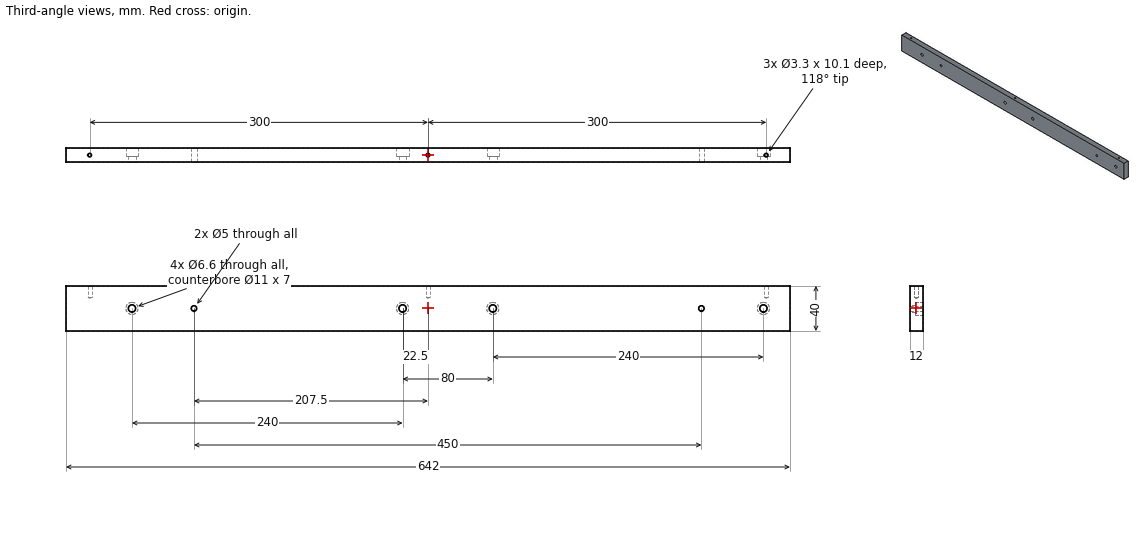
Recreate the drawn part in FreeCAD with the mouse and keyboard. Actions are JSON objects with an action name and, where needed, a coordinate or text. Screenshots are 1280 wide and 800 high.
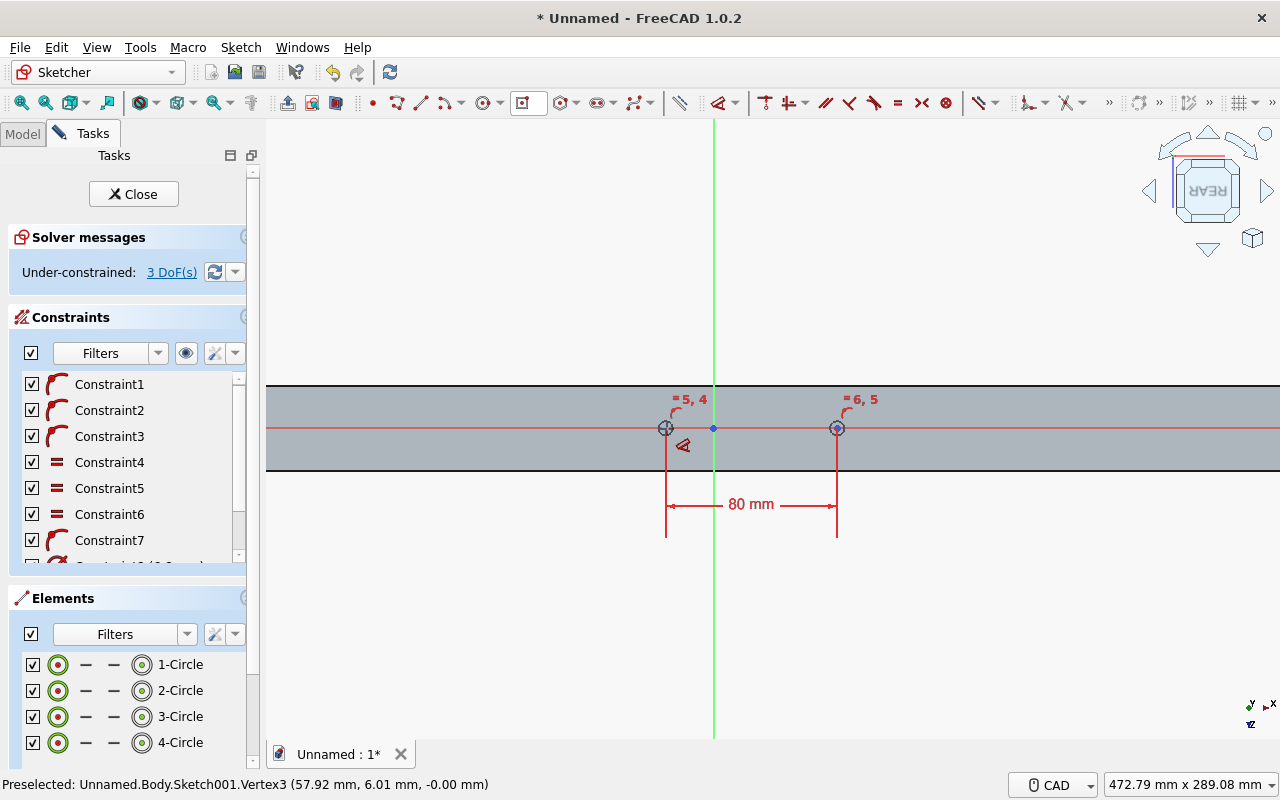
{"action": "left_click", "coordinate": [666, 428]}
{"action": "left_click", "coordinate": [690, 462]}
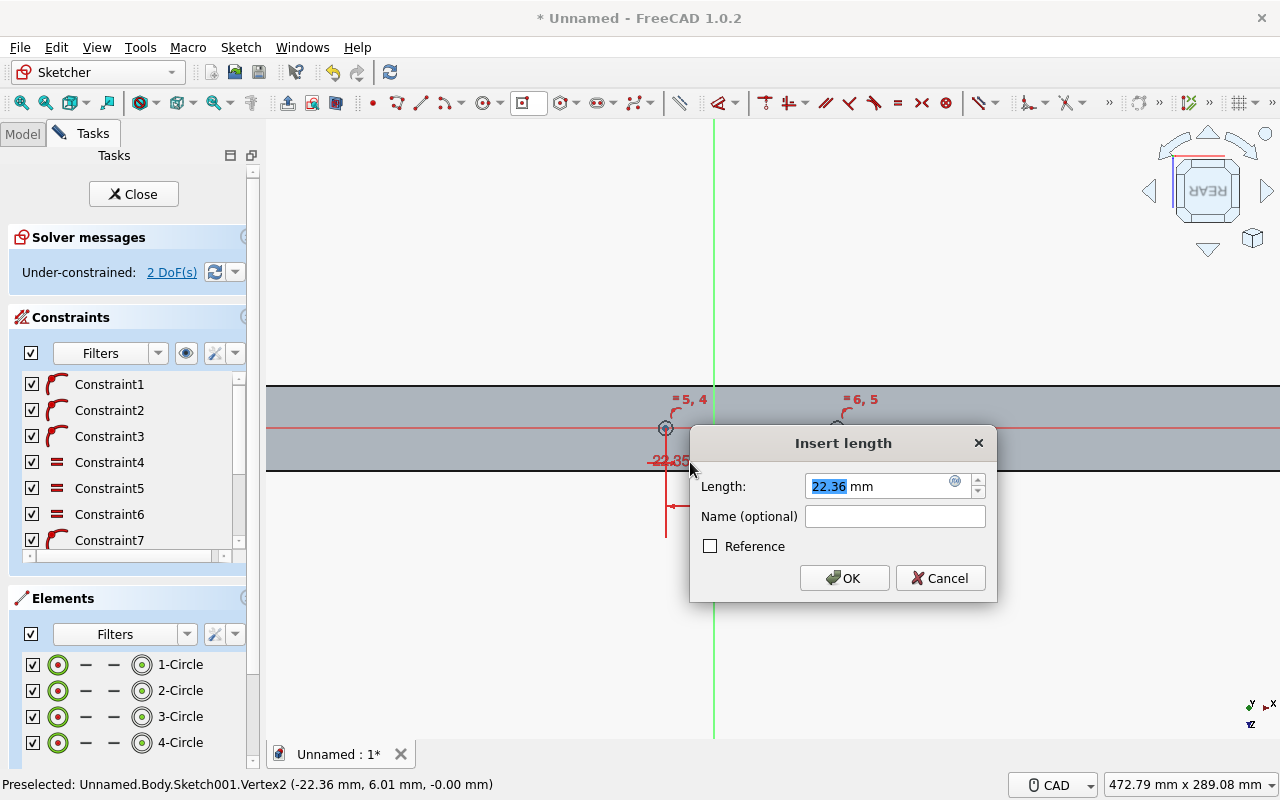
{"action": "type", "text": "22.5"}
{"action": "key", "text": "Return"}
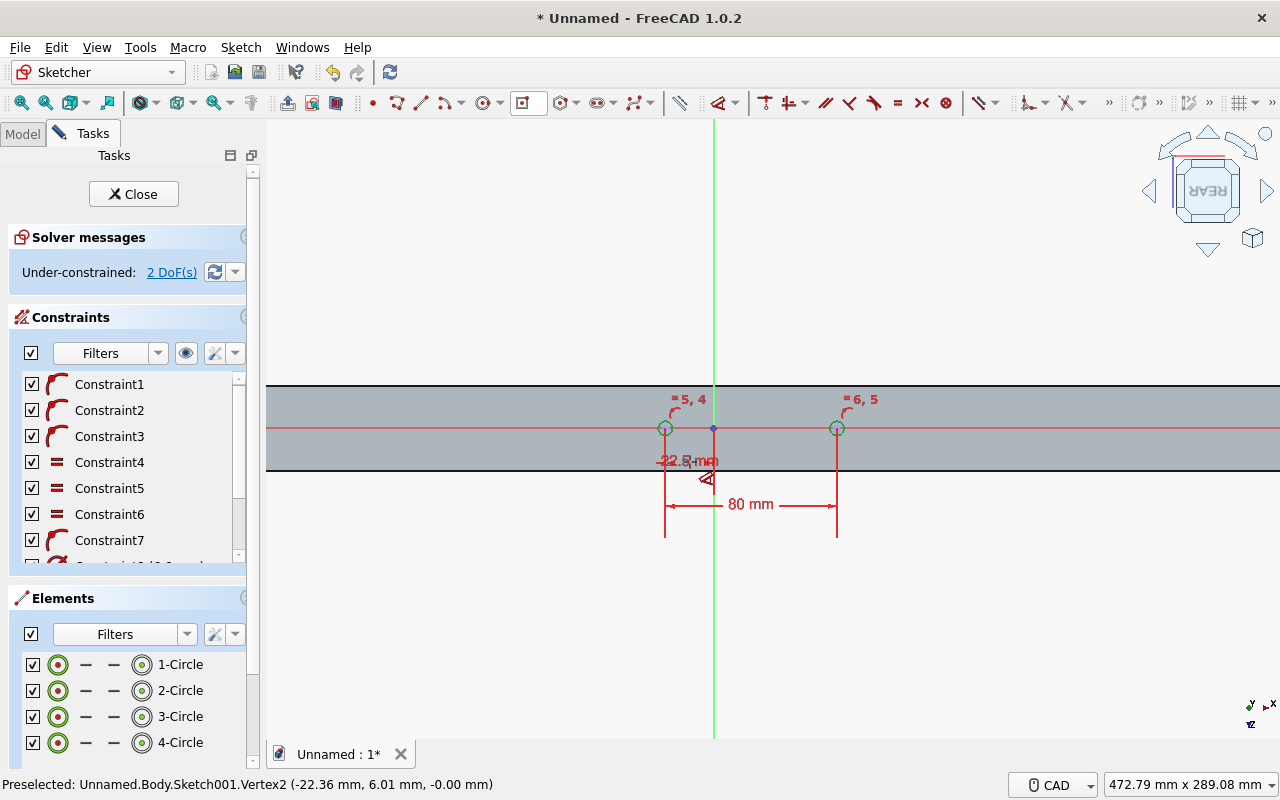
{"action": "scroll", "coordinate": [666, 429], "scroll_direction": "down", "scroll_amount": 4}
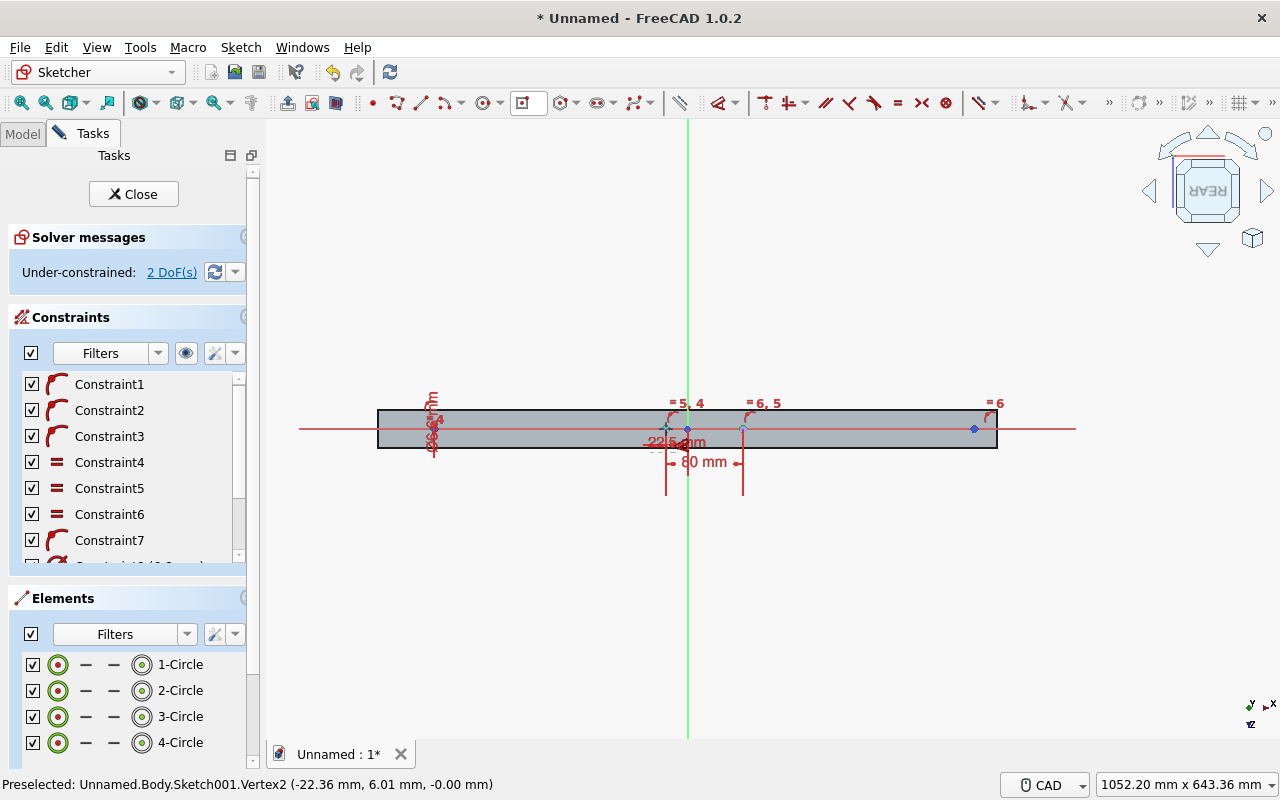
{"action": "left_click", "coordinate": [434, 429]}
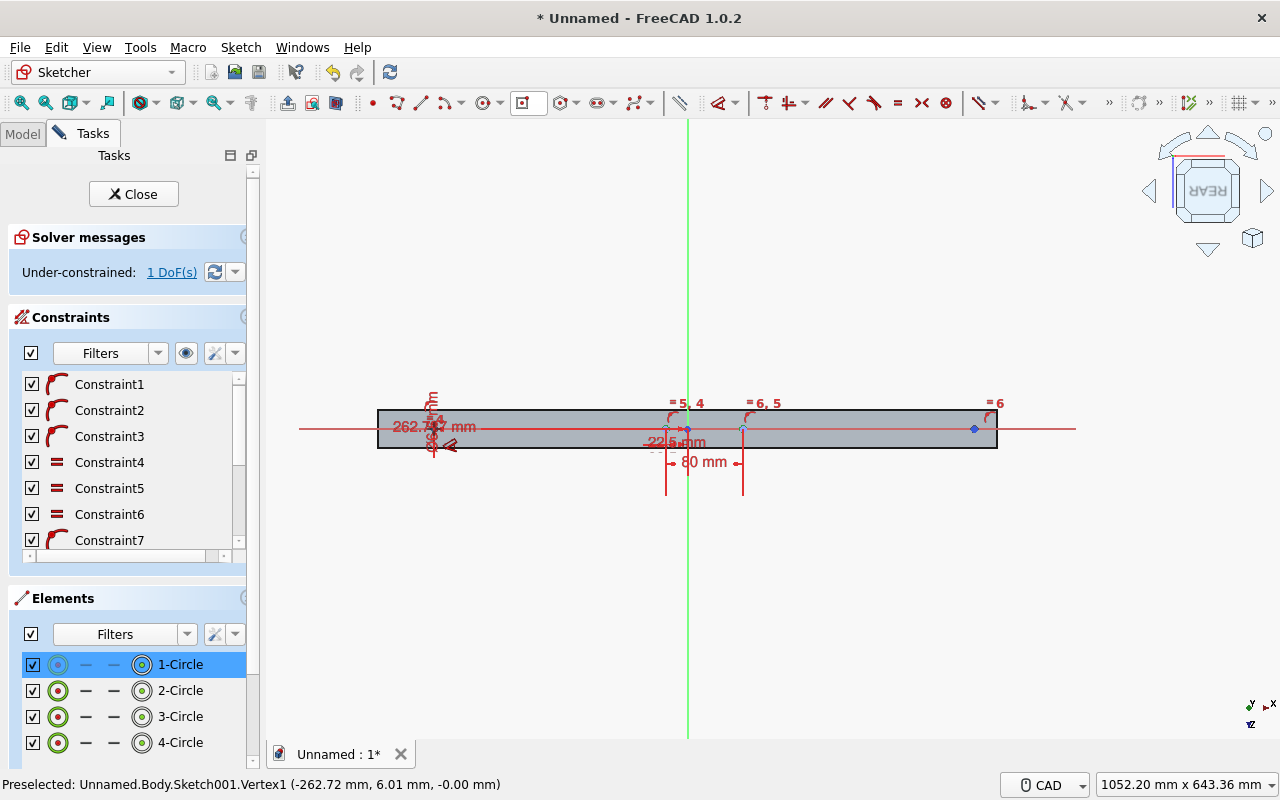
{"action": "left_click", "coordinate": [666, 429]}
{"action": "left_click", "coordinate": [550, 463]}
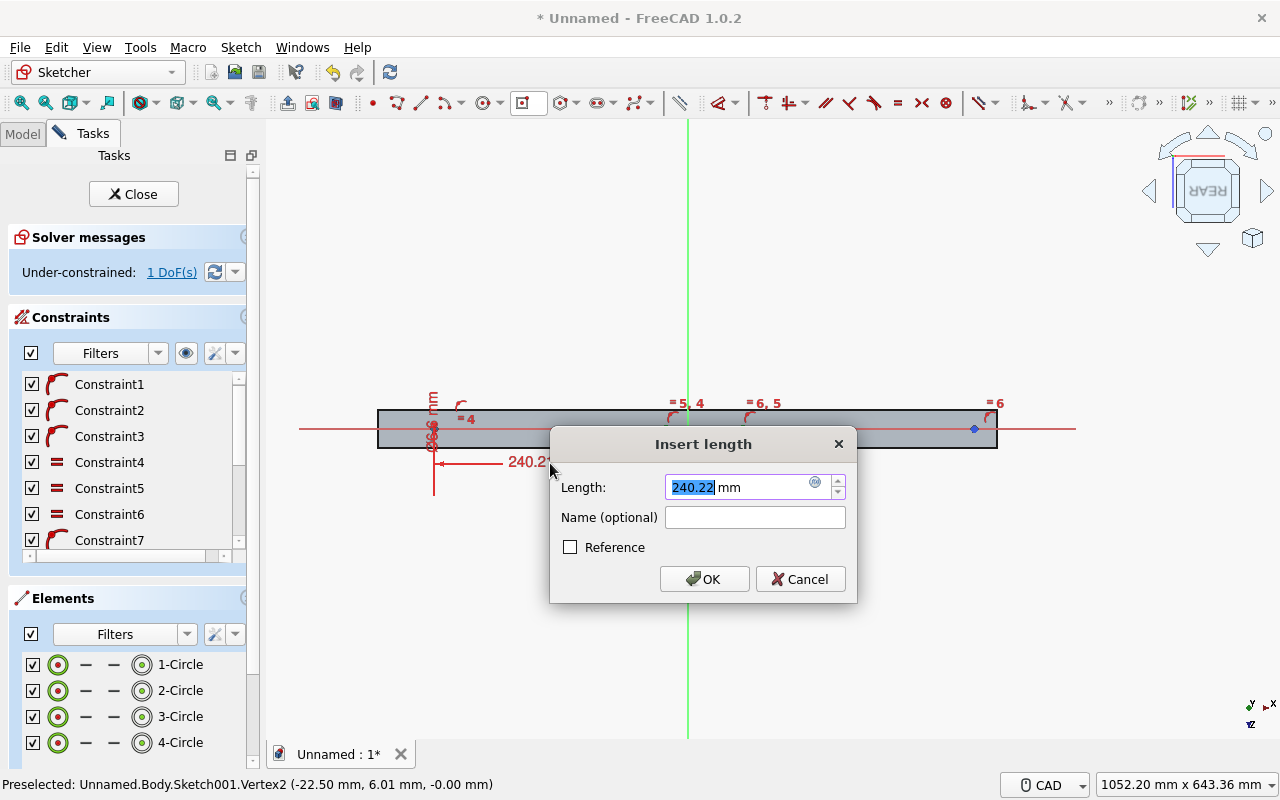
{"action": "type", "text": "240"}
{"action": "key", "text": "Return"}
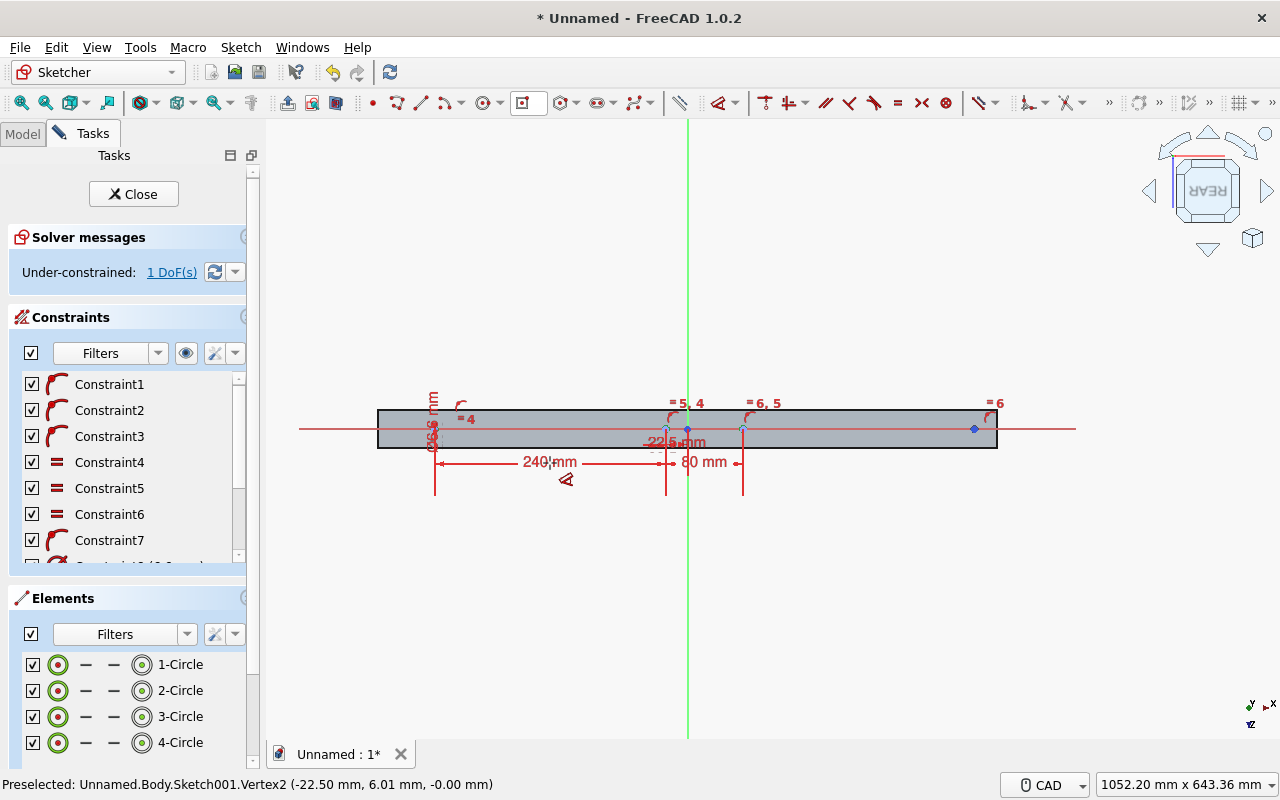
{"action": "left_click", "coordinate": [743, 429]}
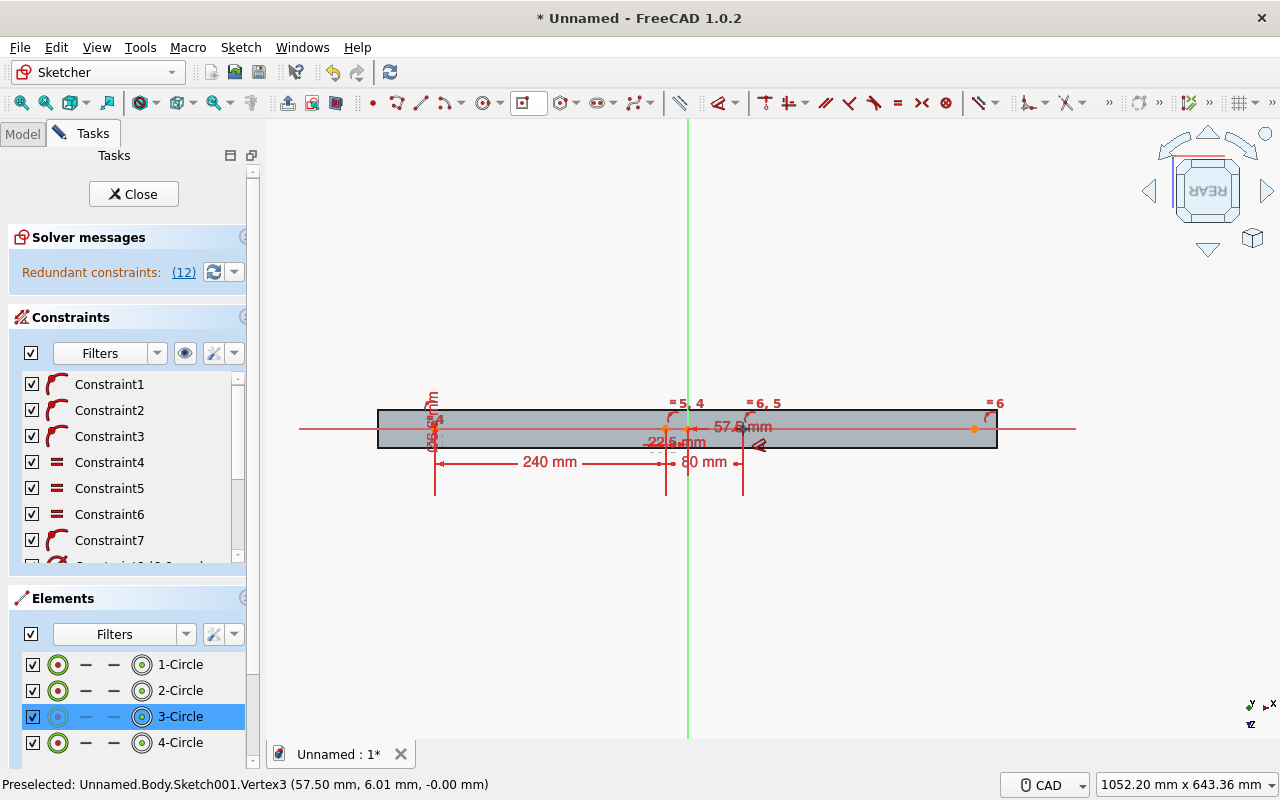
{"action": "left_click", "coordinate": [974, 429]}
{"action": "left_click", "coordinate": [859, 463]}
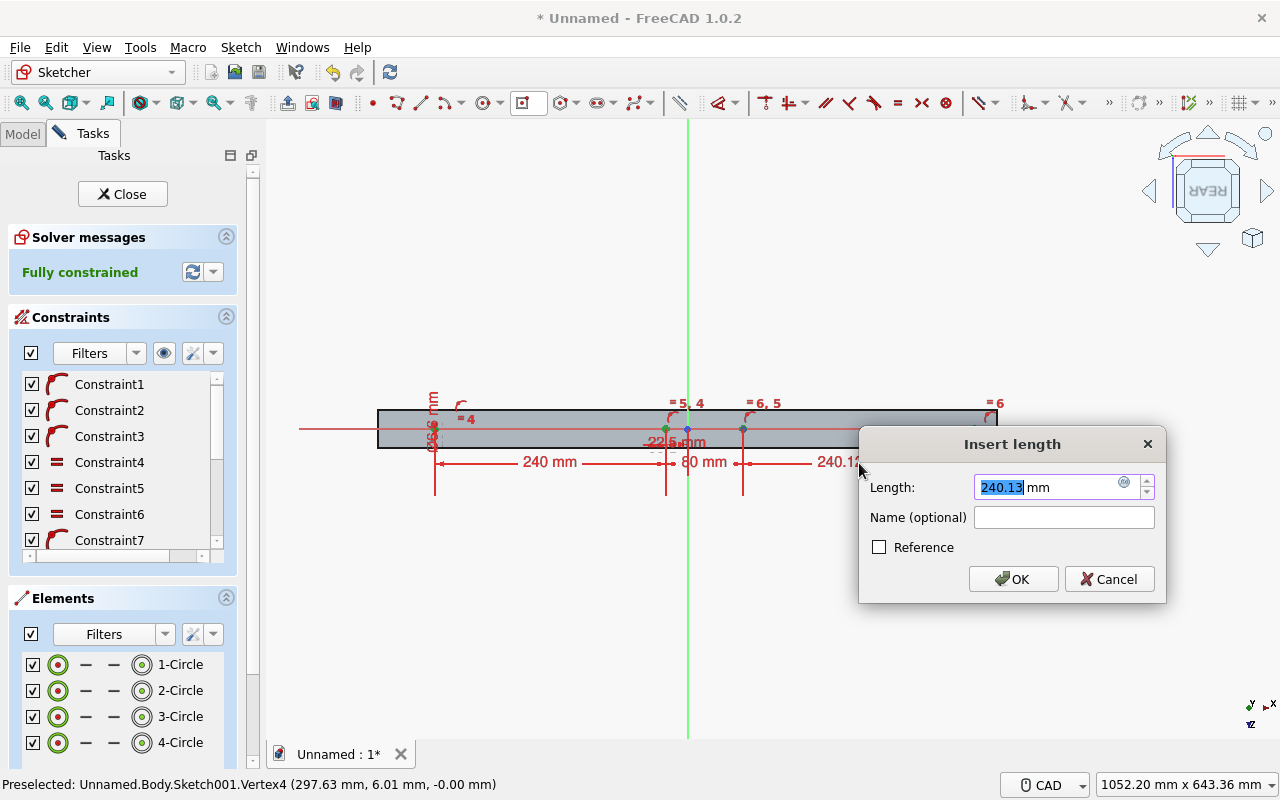
{"action": "type", "text": "240"}
{"action": "key", "text": "Return"}
{"action": "key", "text": "Escape"}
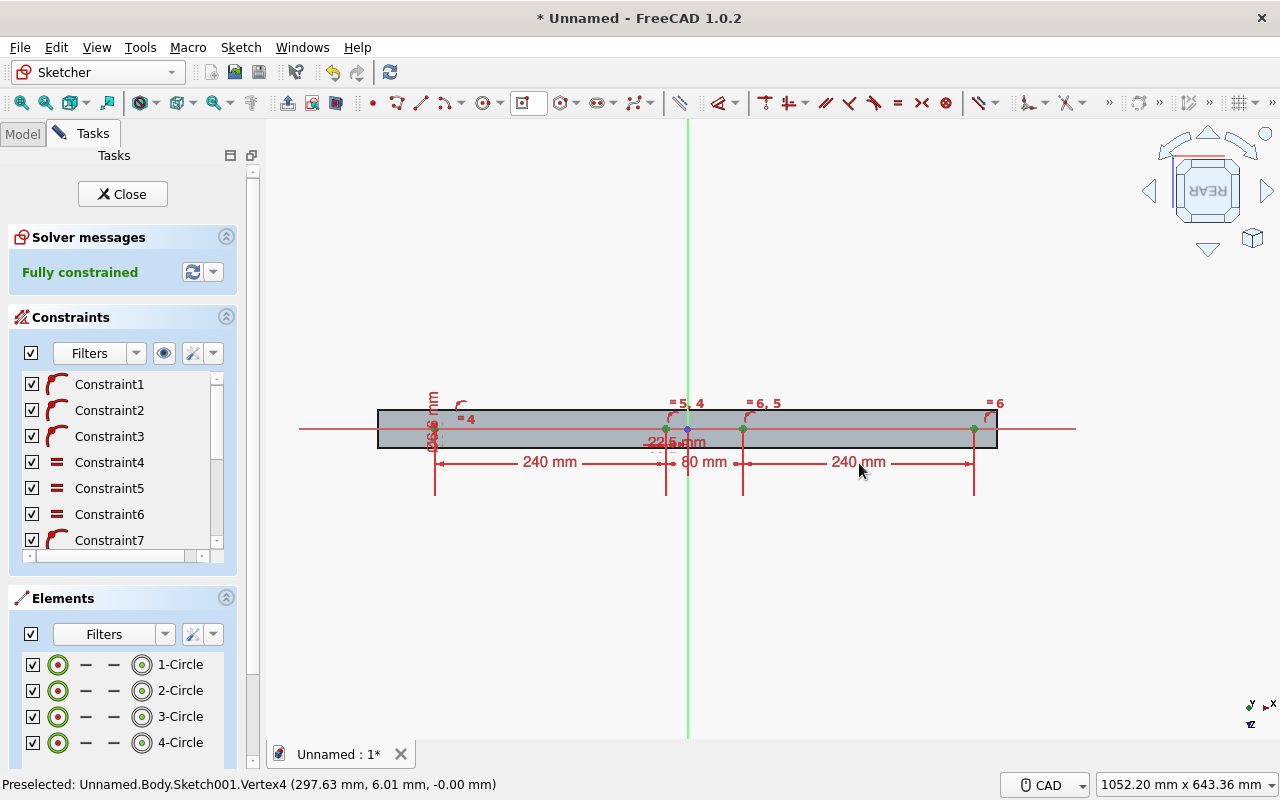
{"action": "left_click", "coordinate": [123, 194]}